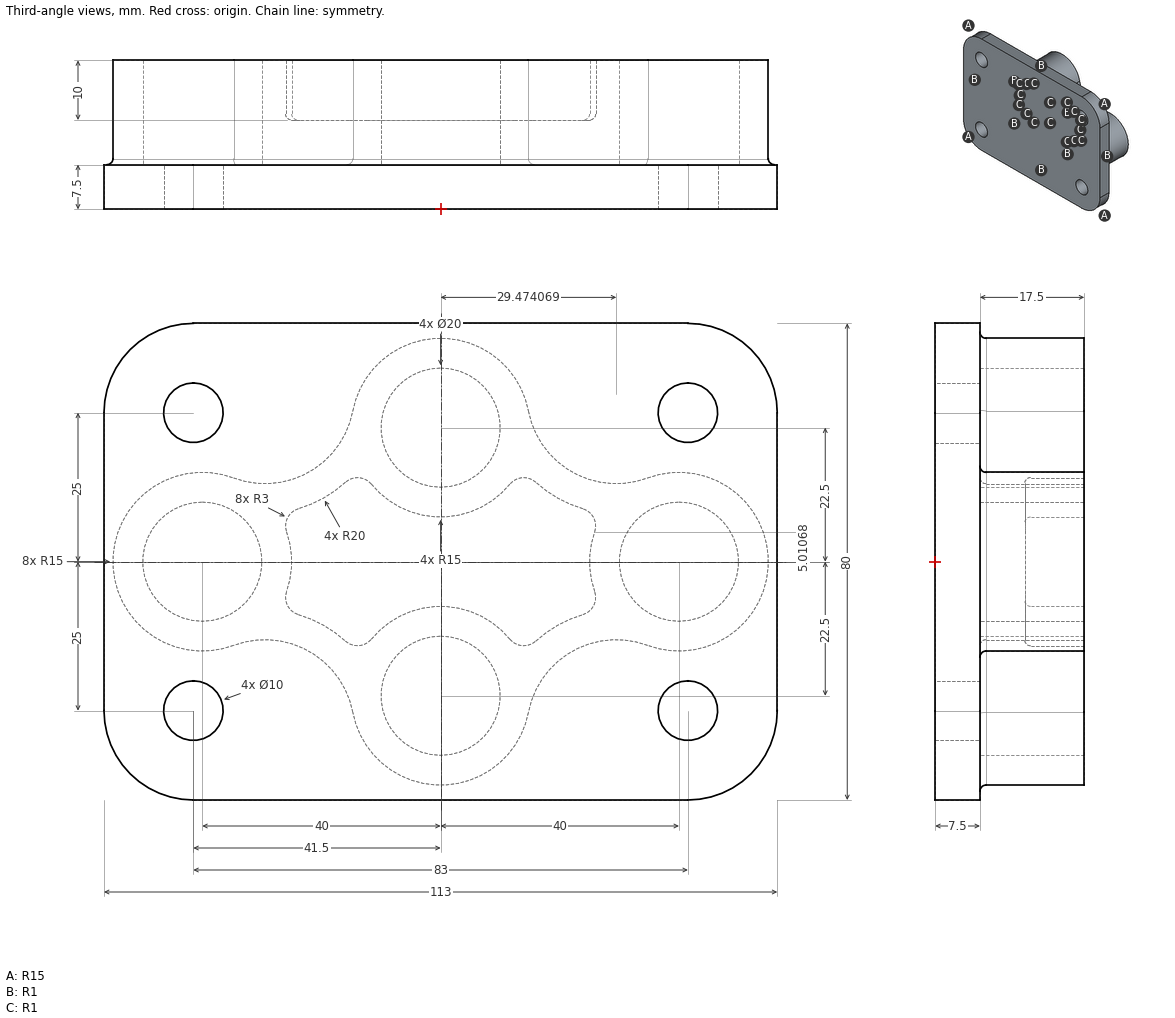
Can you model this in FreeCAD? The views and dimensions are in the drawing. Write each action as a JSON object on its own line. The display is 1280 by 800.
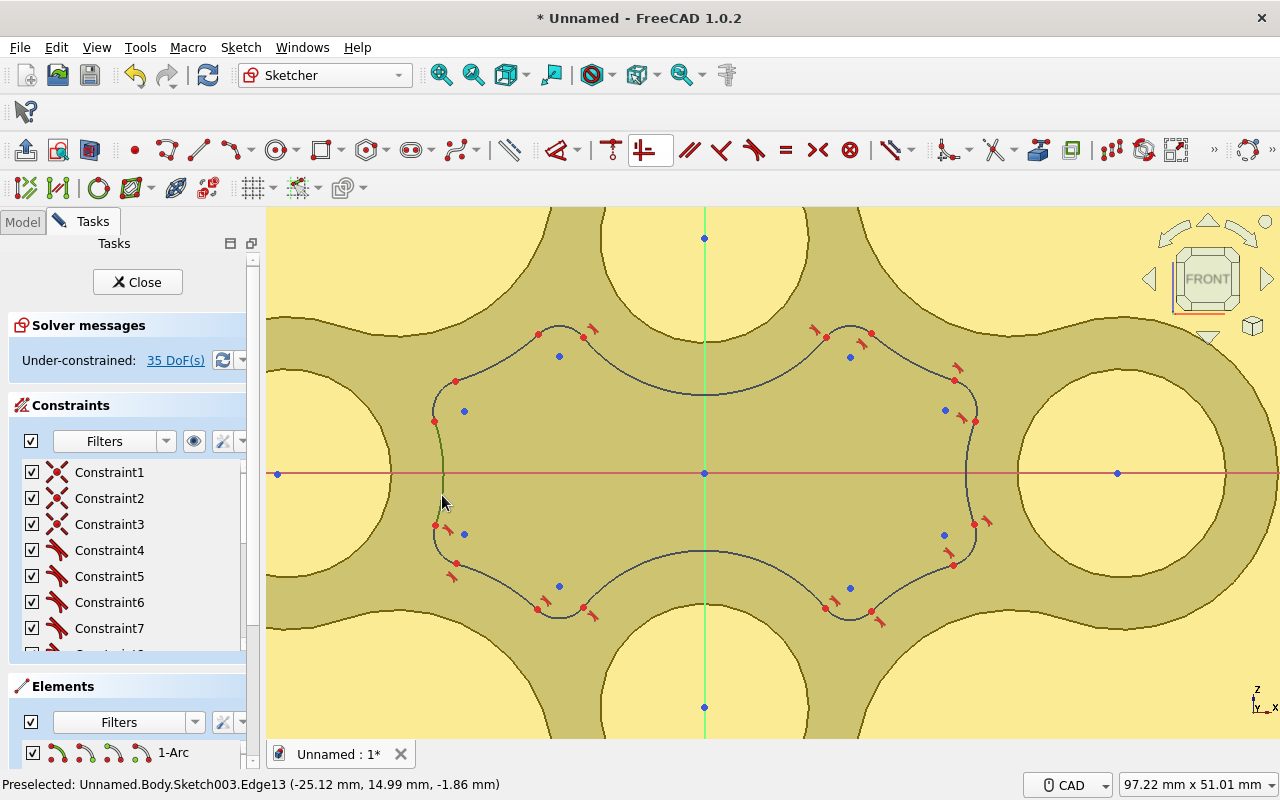
{"action": "left_click", "coordinate": [442, 389]}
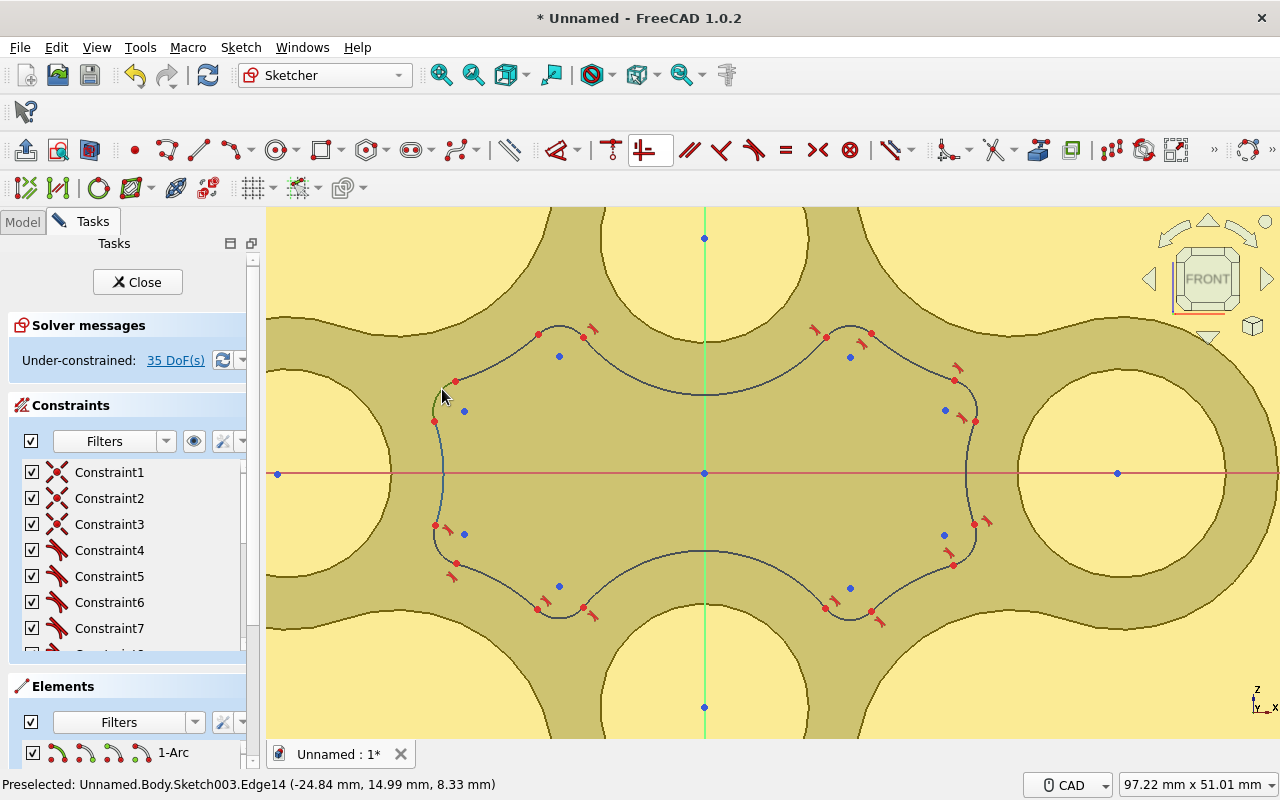
{"action": "key", "text": "t"}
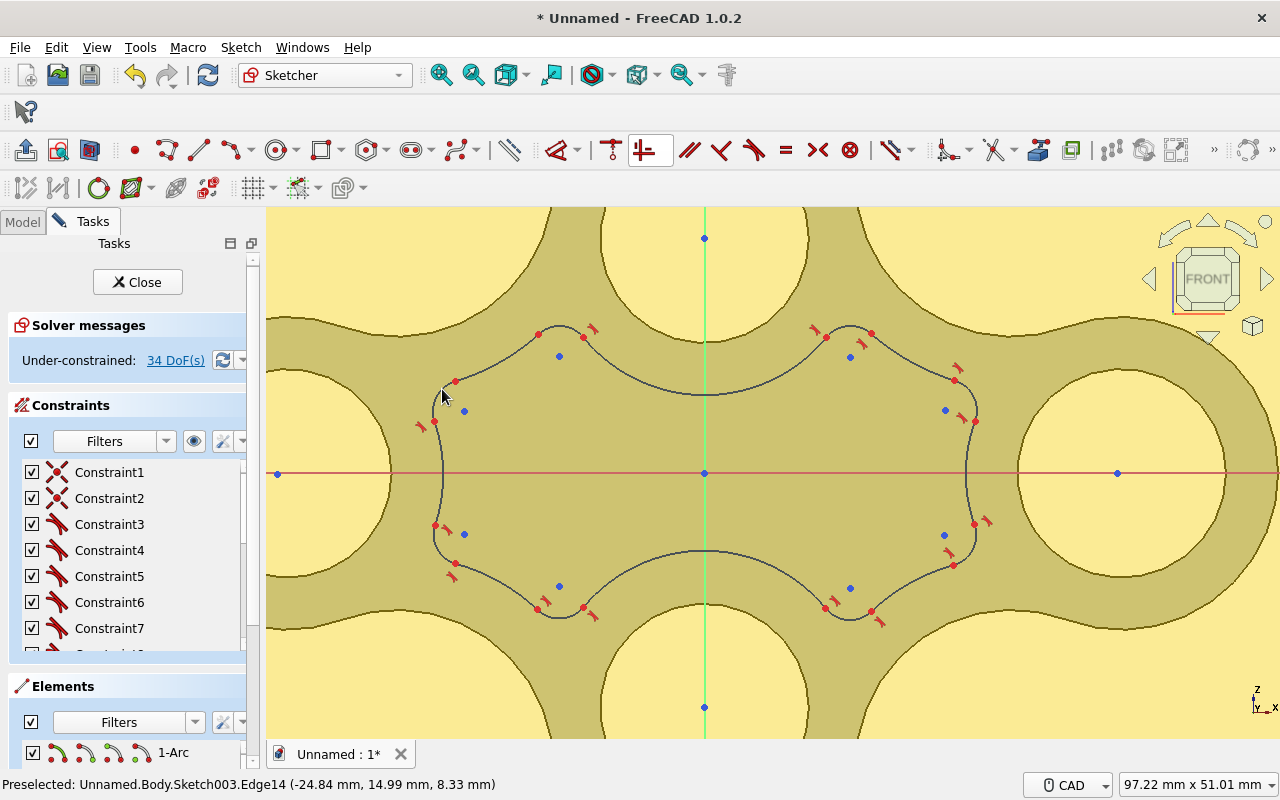
{"action": "left_click", "coordinate": [442, 389]}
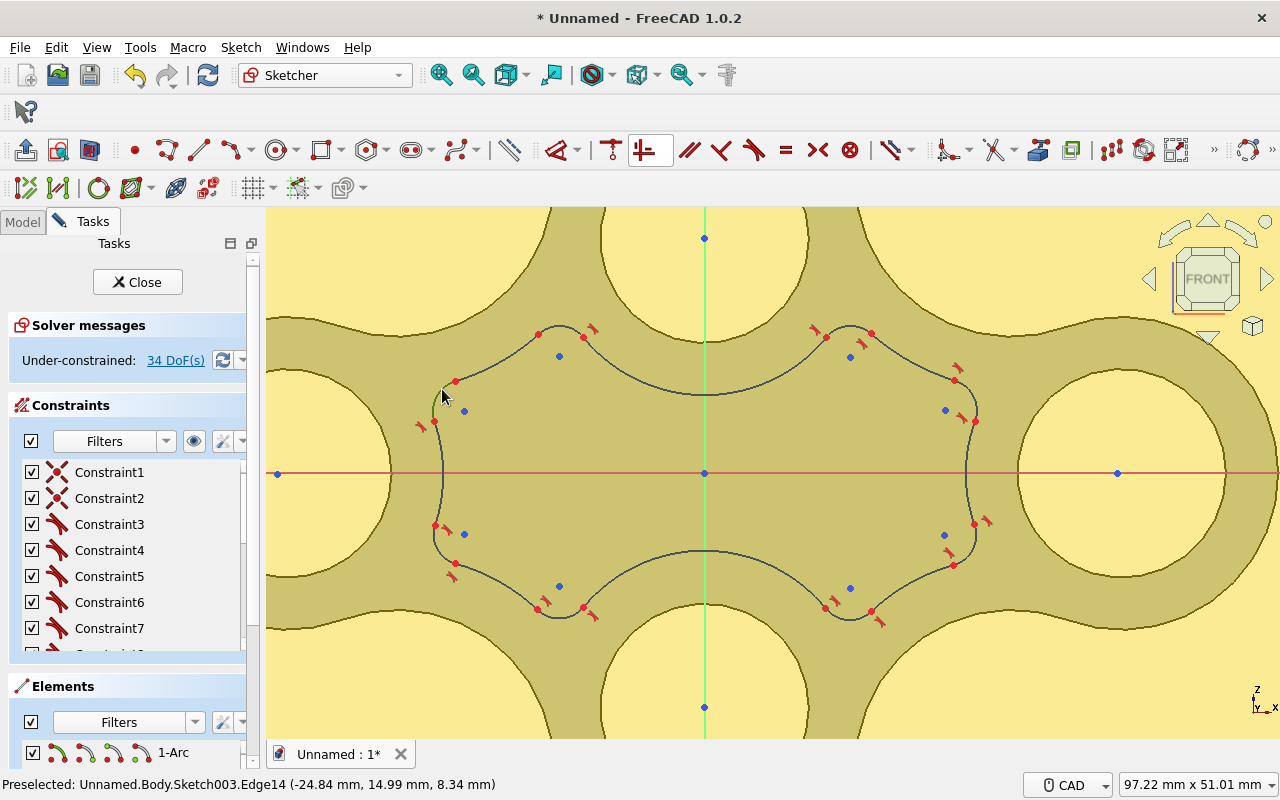
{"action": "left_click", "coordinate": [482, 371]}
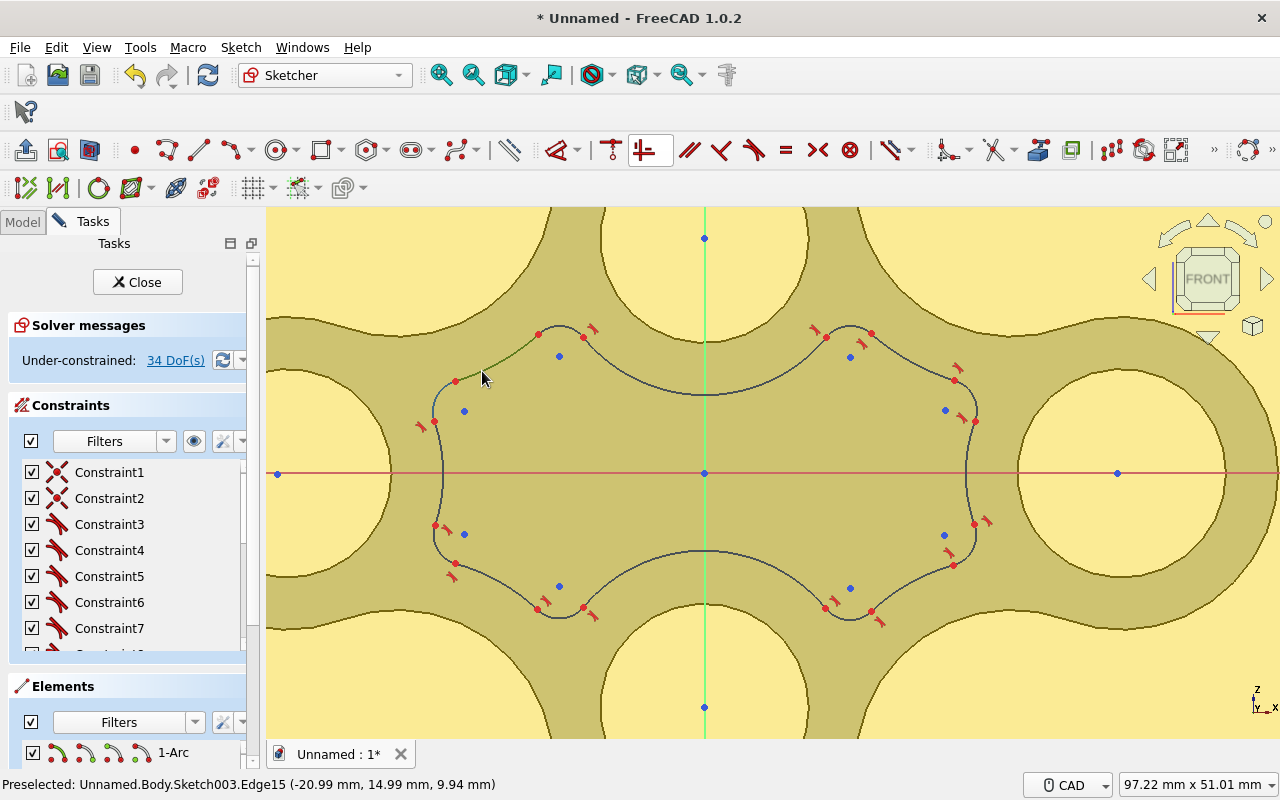
{"action": "left_click", "coordinate": [754, 150]}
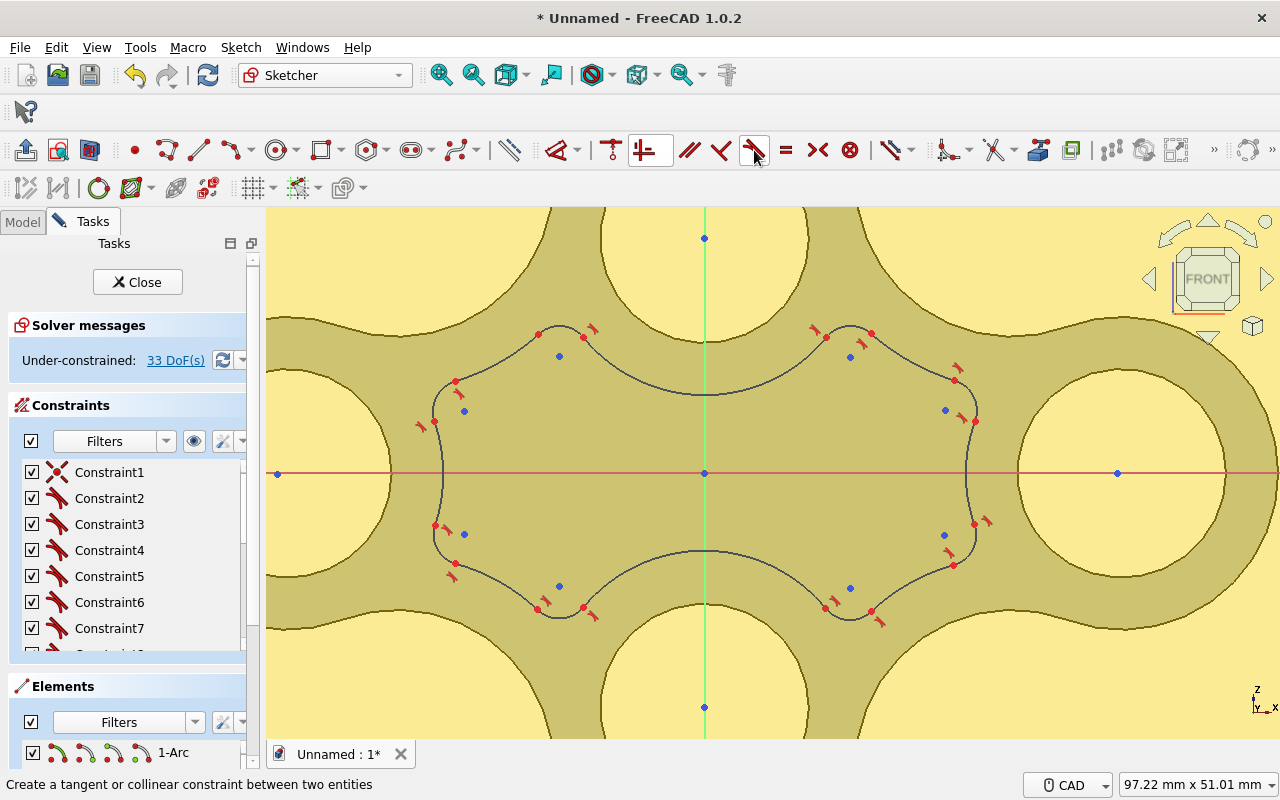
{"action": "left_click", "coordinate": [482, 371]}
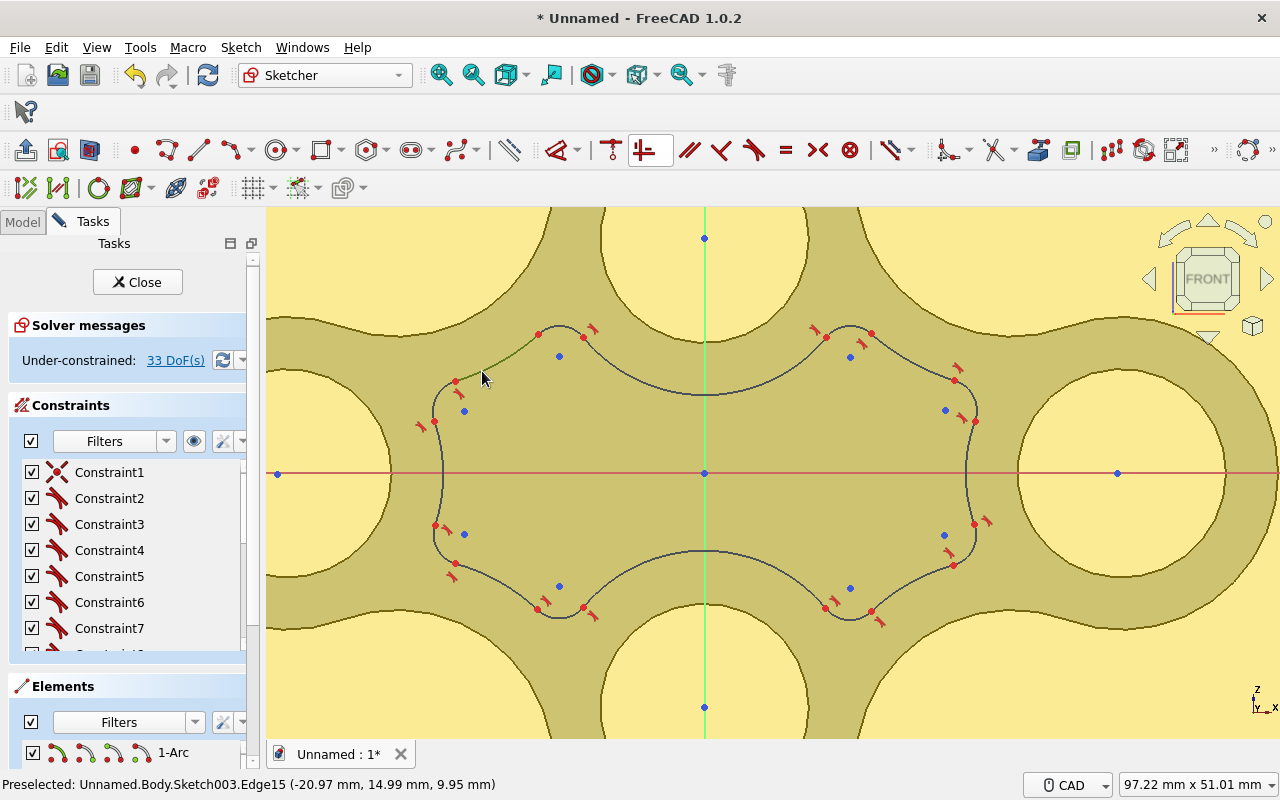
{"action": "left_click", "coordinate": [571, 328]}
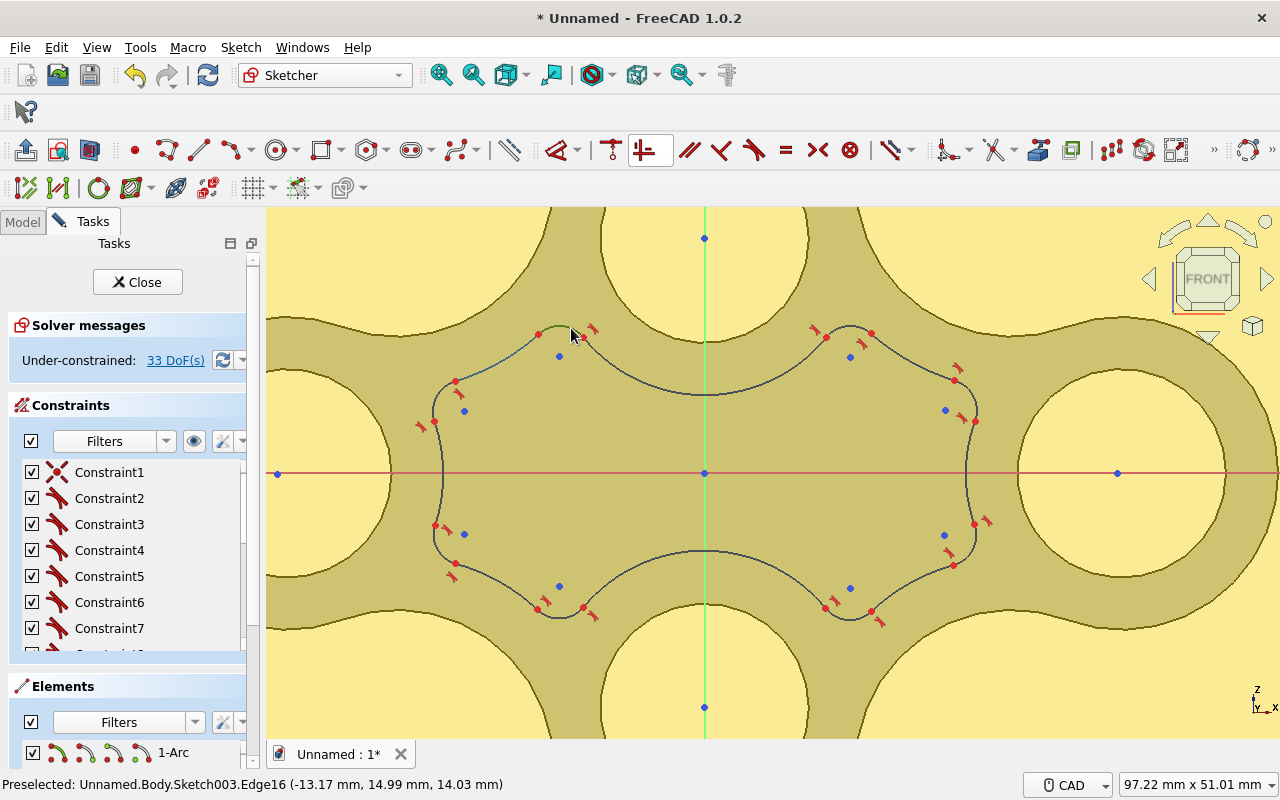
{"action": "key", "text": "t"}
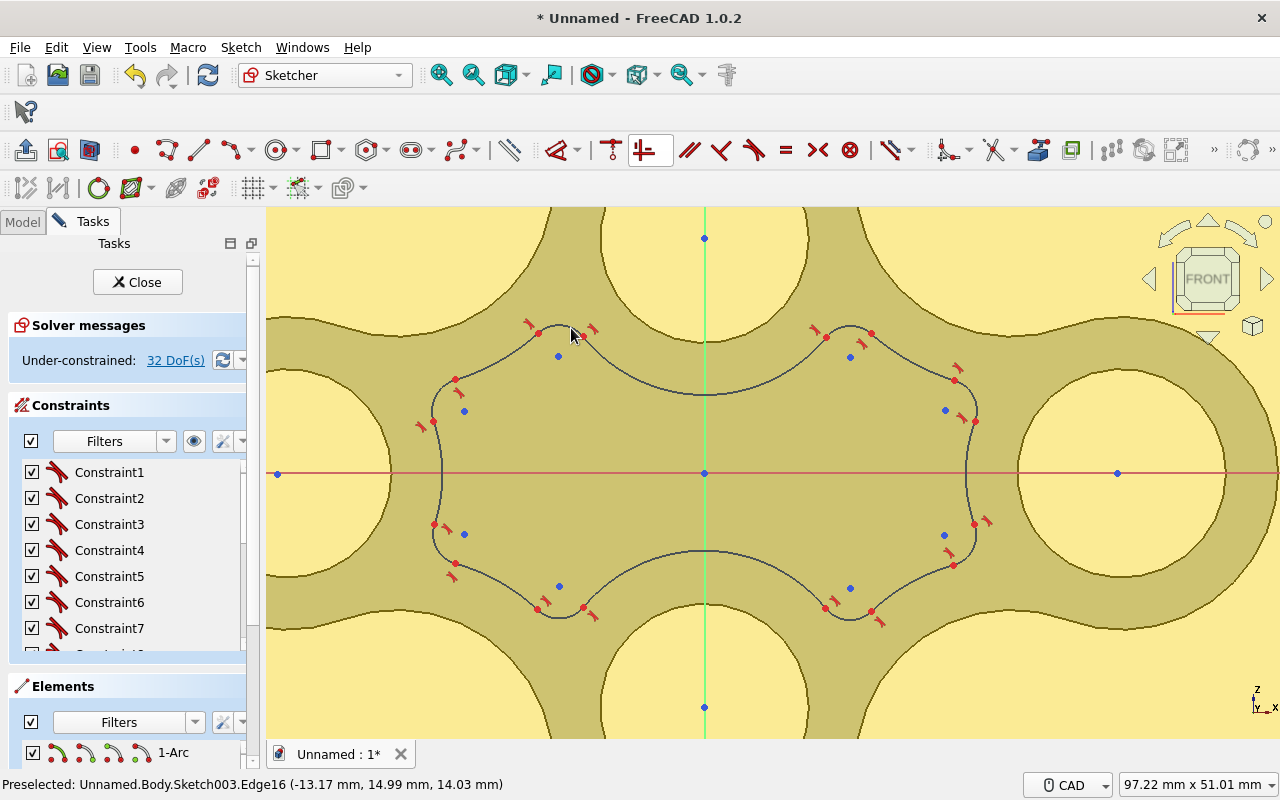
{"action": "left_click", "coordinate": [858, 327]}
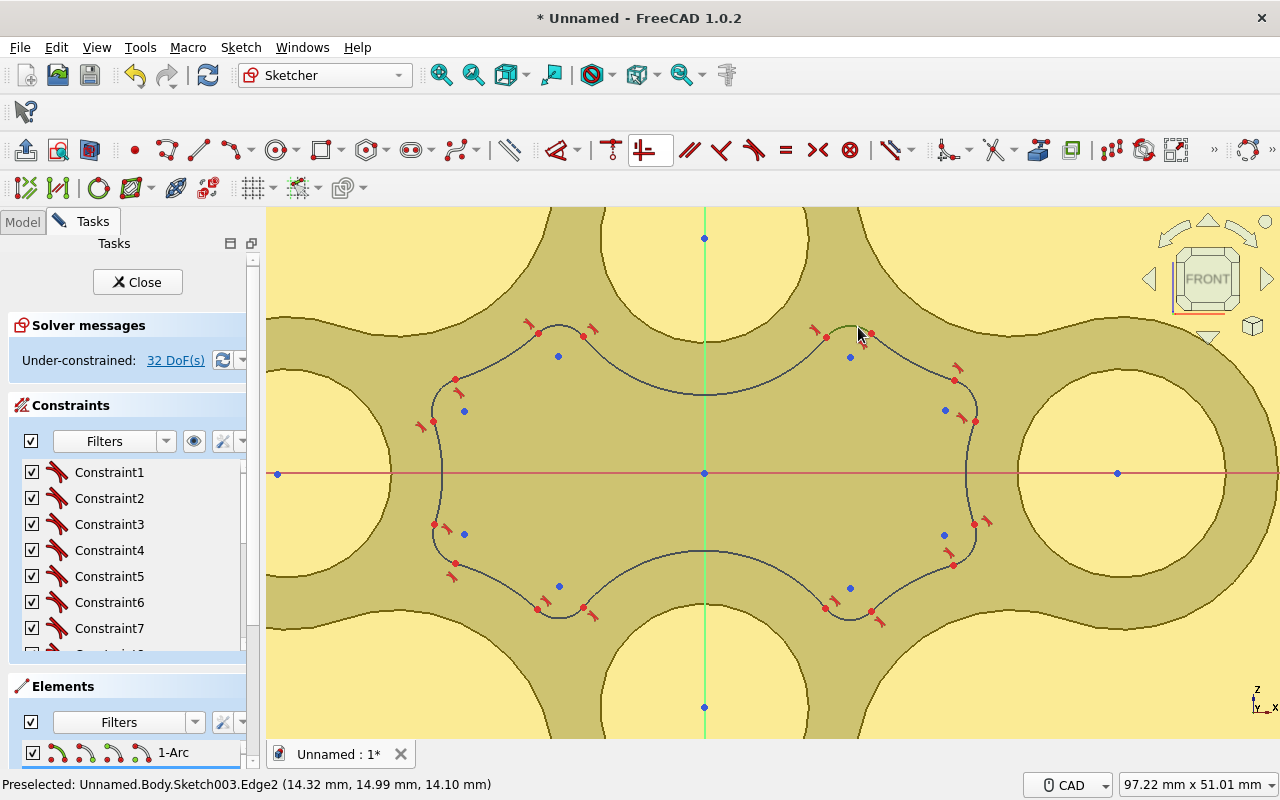
{"action": "left_click", "coordinate": [977, 407]}